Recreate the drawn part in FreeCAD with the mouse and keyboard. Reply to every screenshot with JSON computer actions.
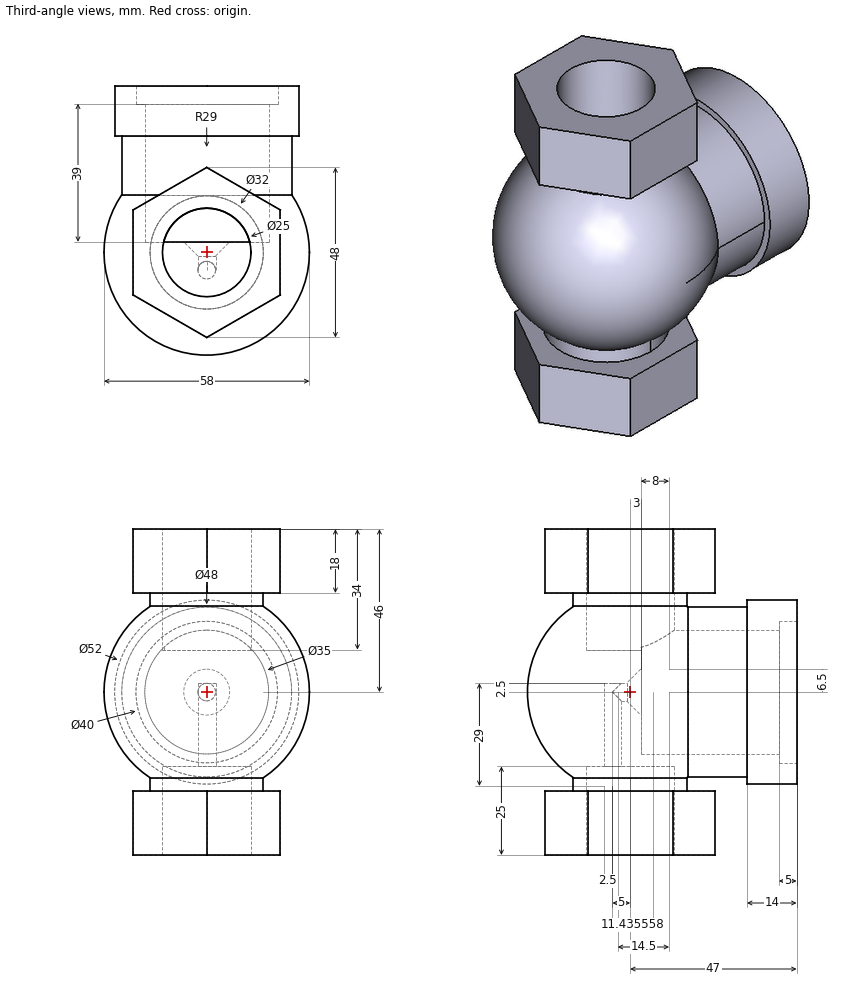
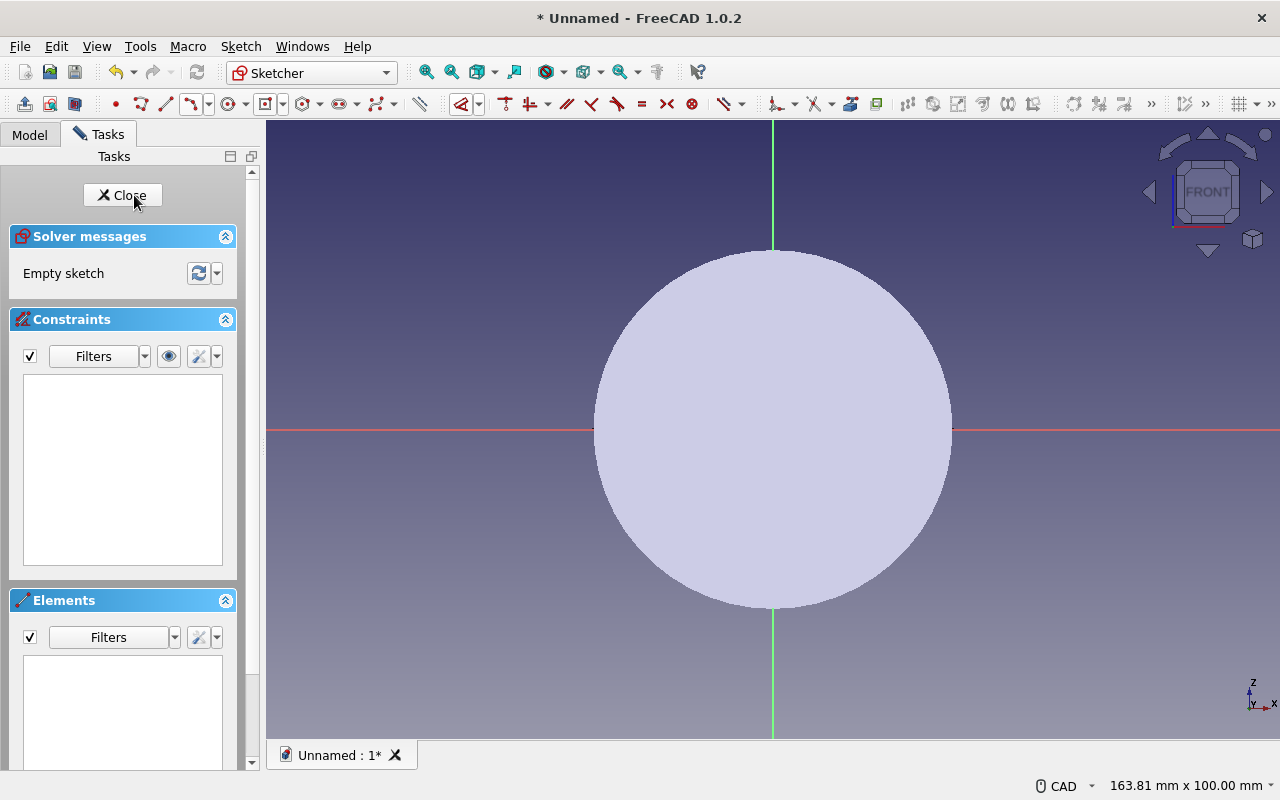
{"action": "left_click", "coordinate": [75, 104]}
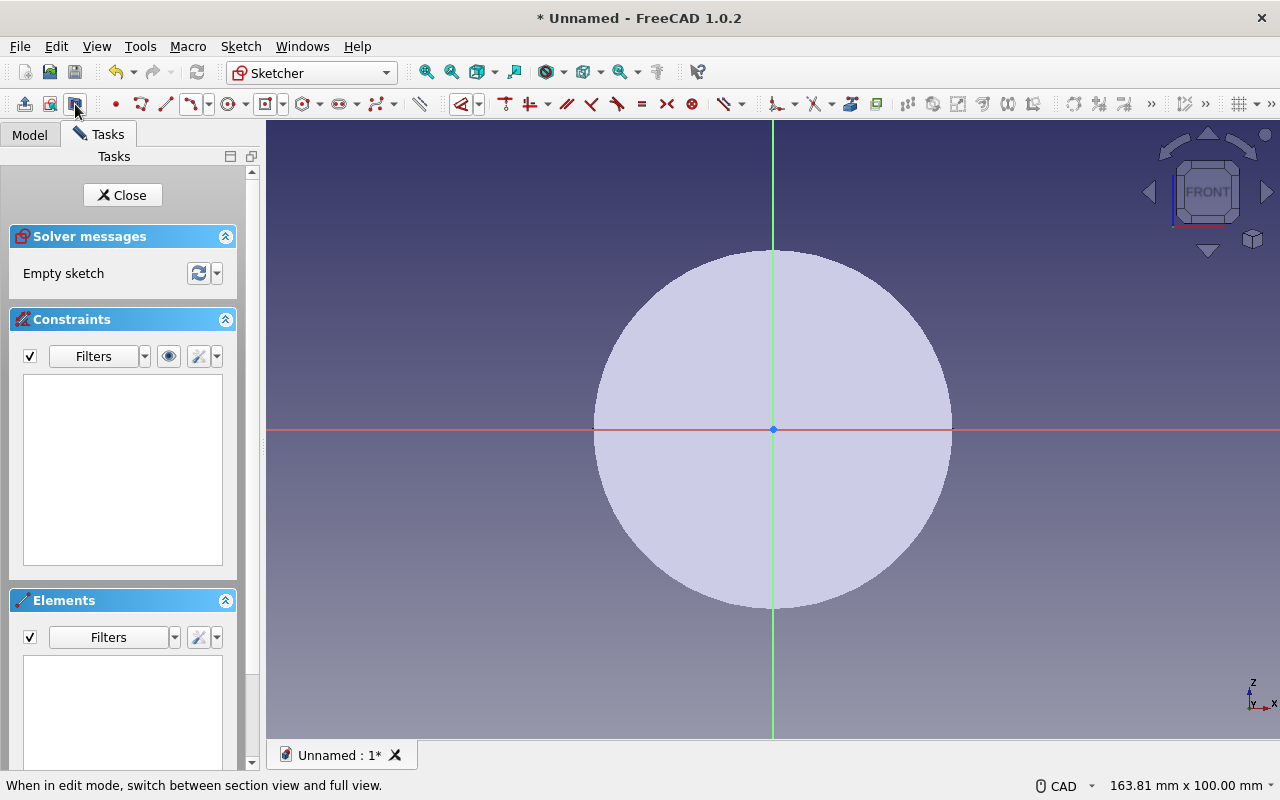
{"action": "left_click", "coordinate": [228, 104]}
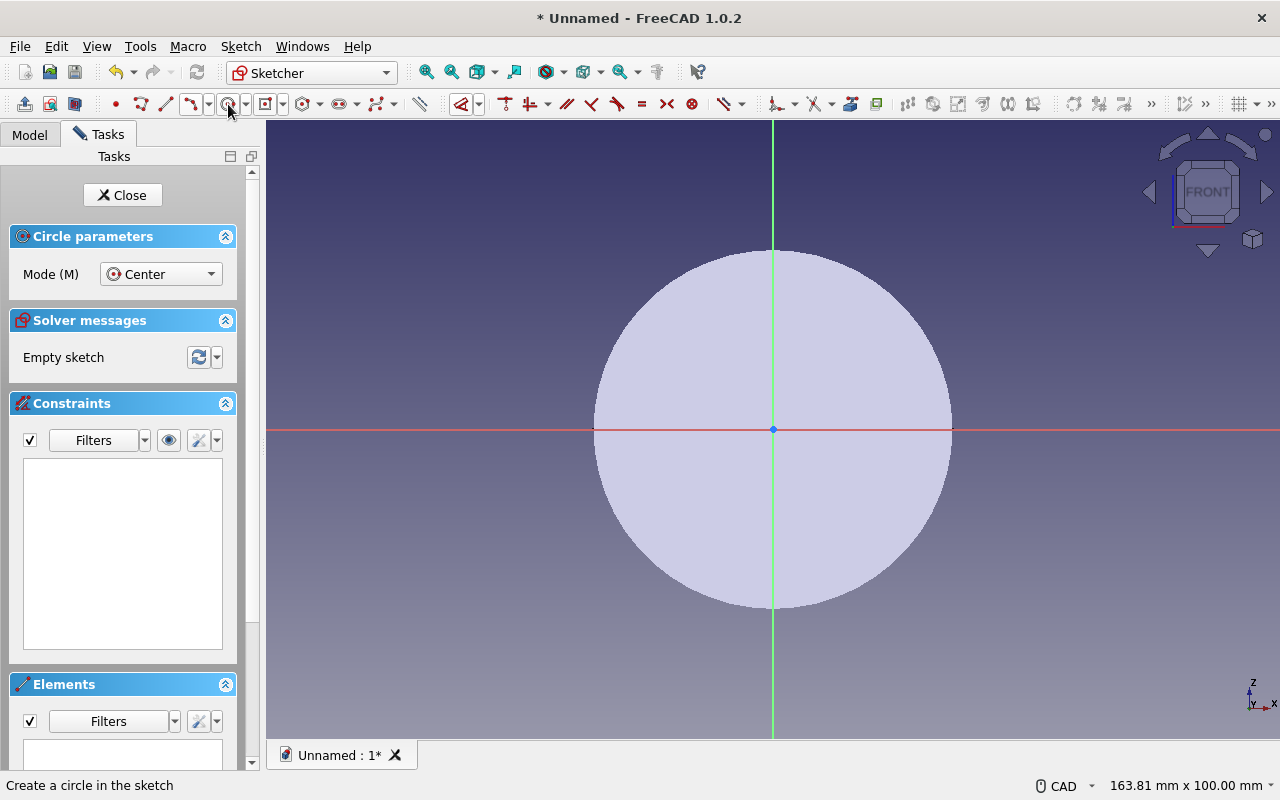
{"action": "left_click", "coordinate": [773, 430]}
{"action": "left_click", "coordinate": [878, 324]}
{"action": "key", "text": "Escape"}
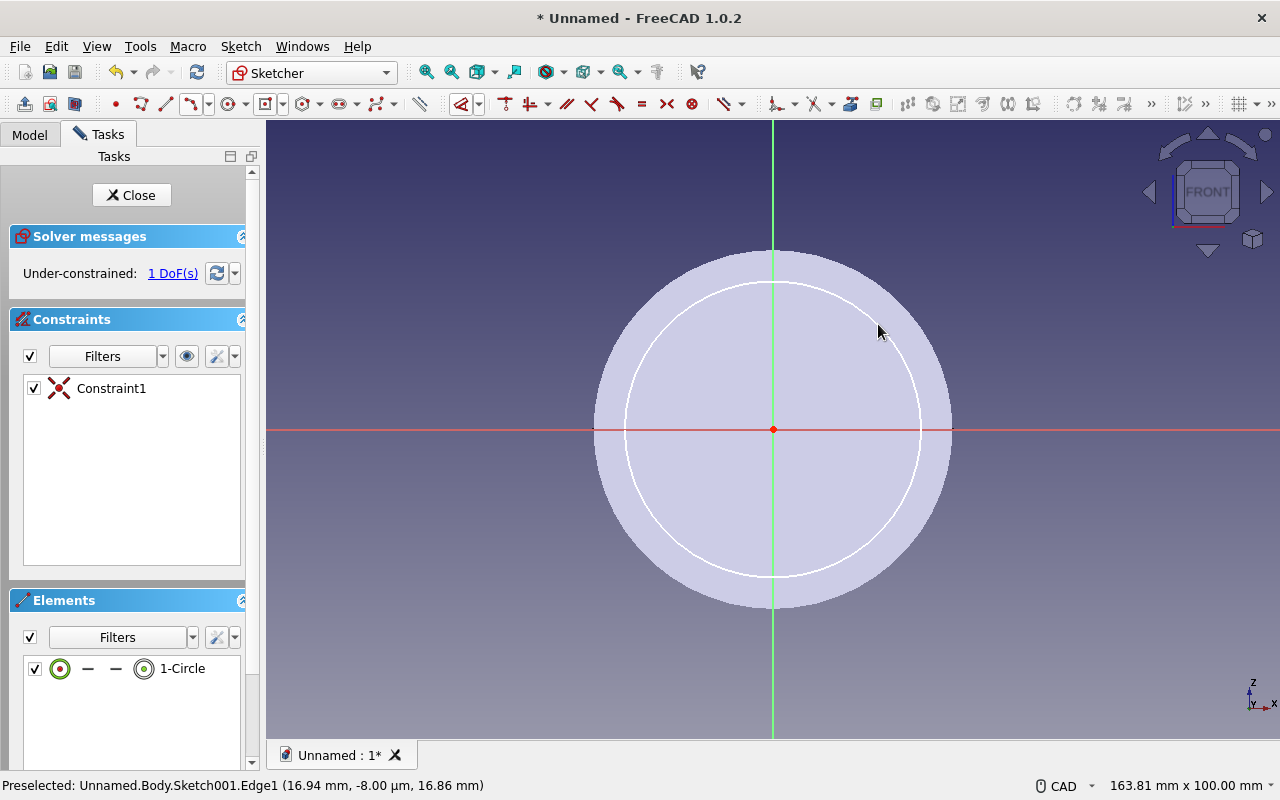
{"action": "left_click", "coordinate": [877, 324]}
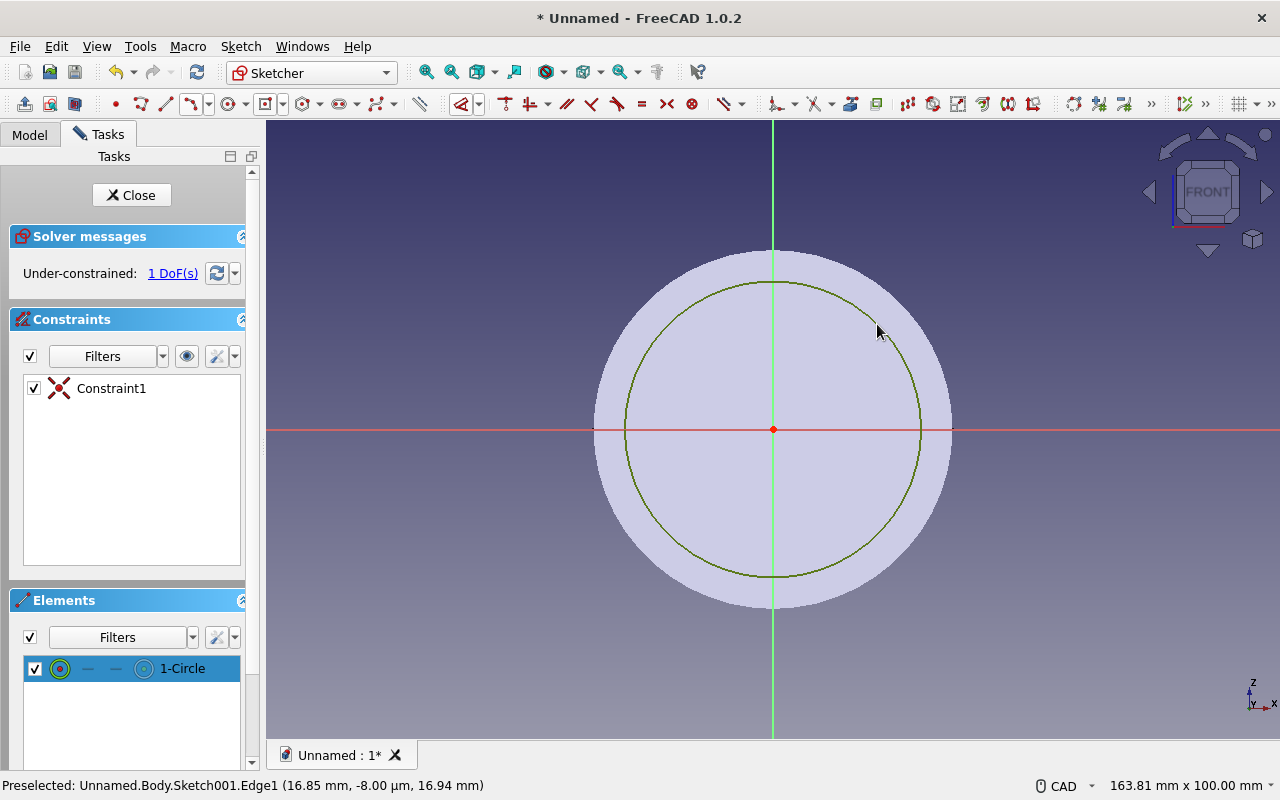
{"action": "key", "text": "k o"}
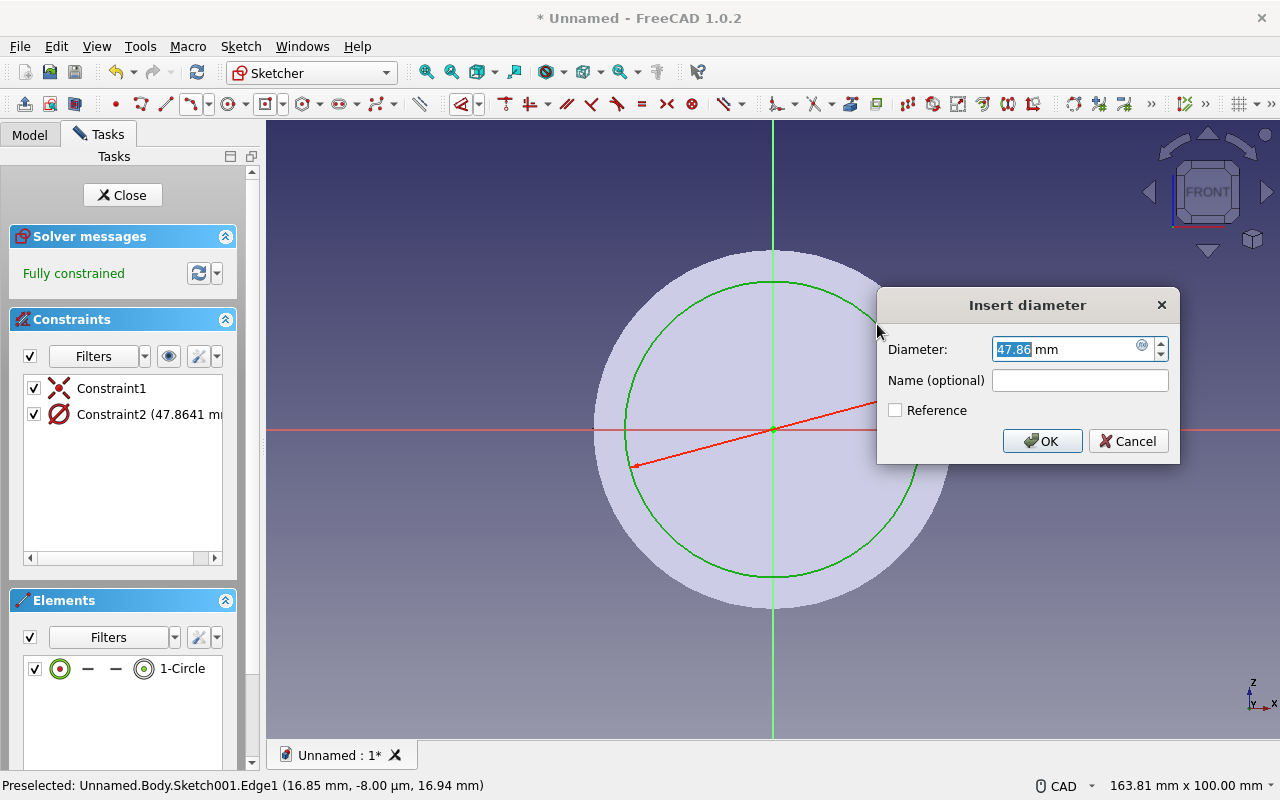
{"action": "type", "text": "48"}
{"action": "key", "text": "Return"}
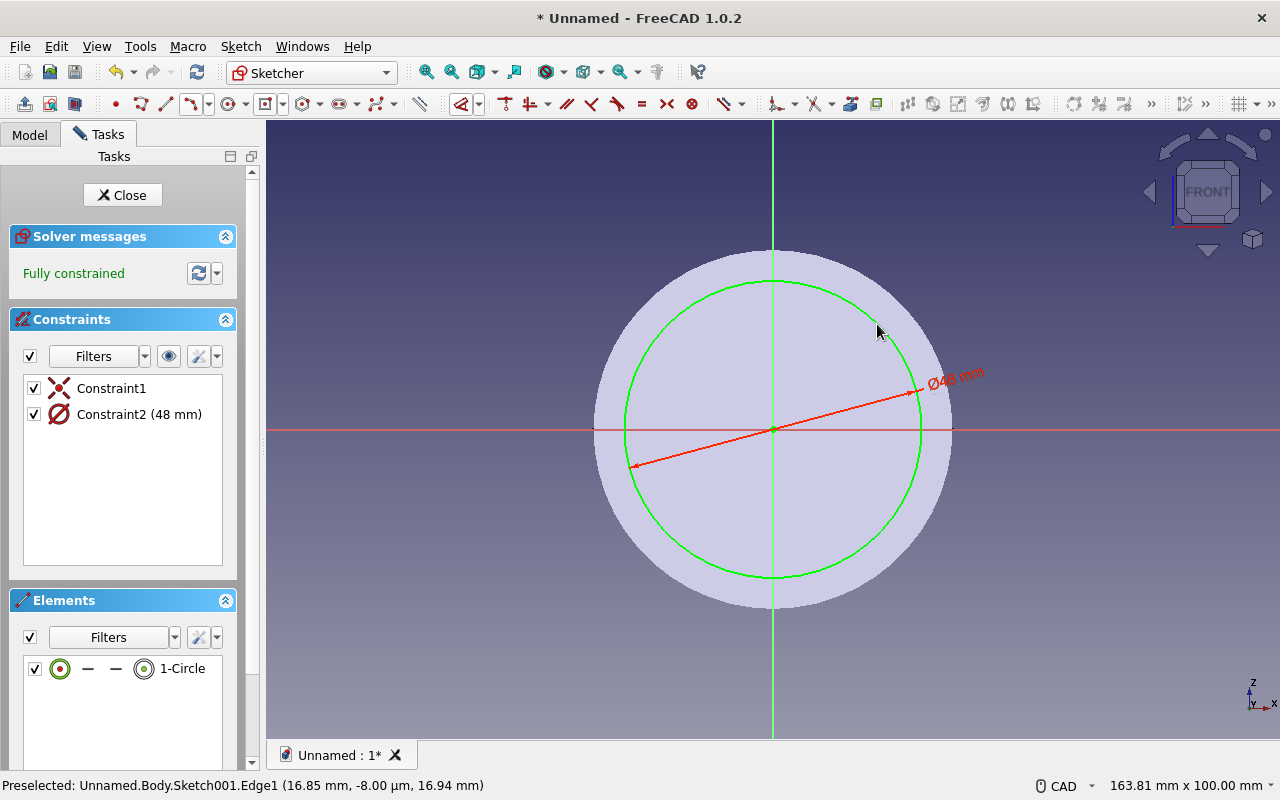
{"action": "left_click", "coordinate": [123, 195]}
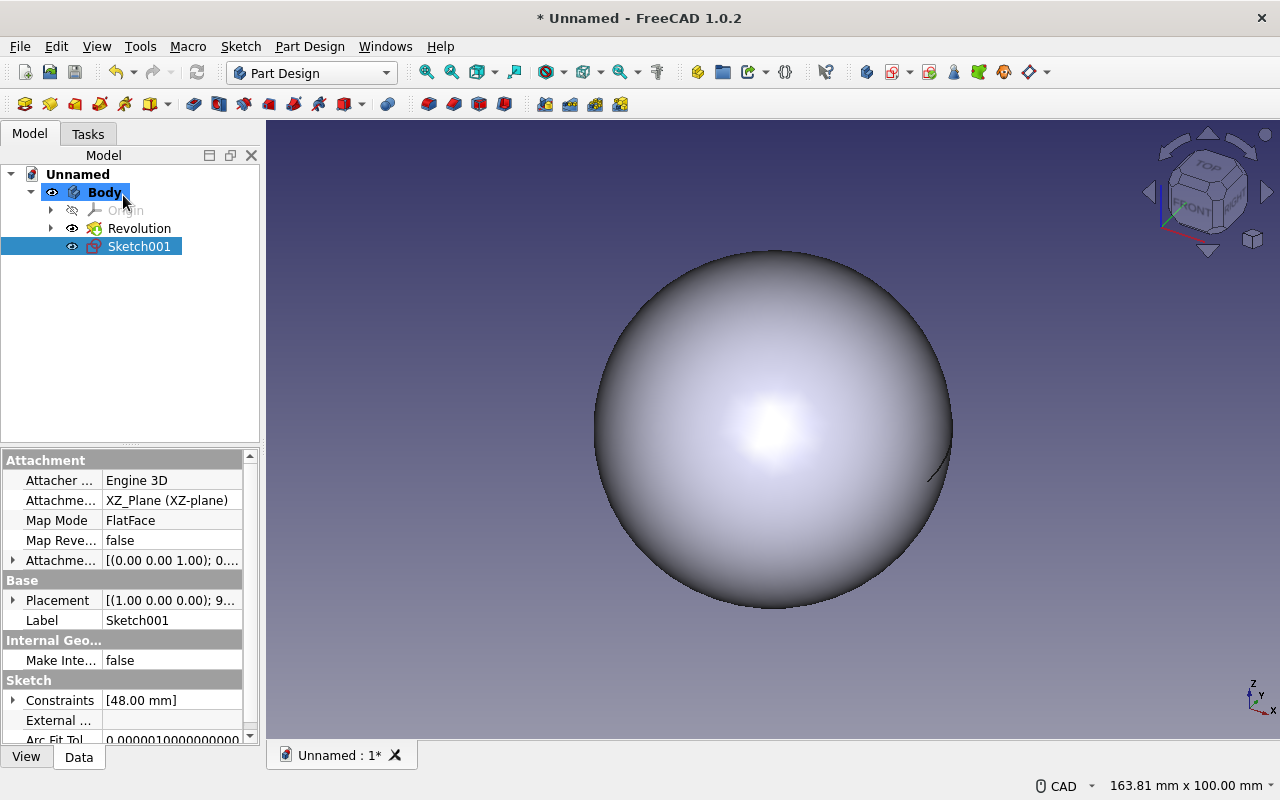
{"action": "left_click", "coordinate": [25, 104]}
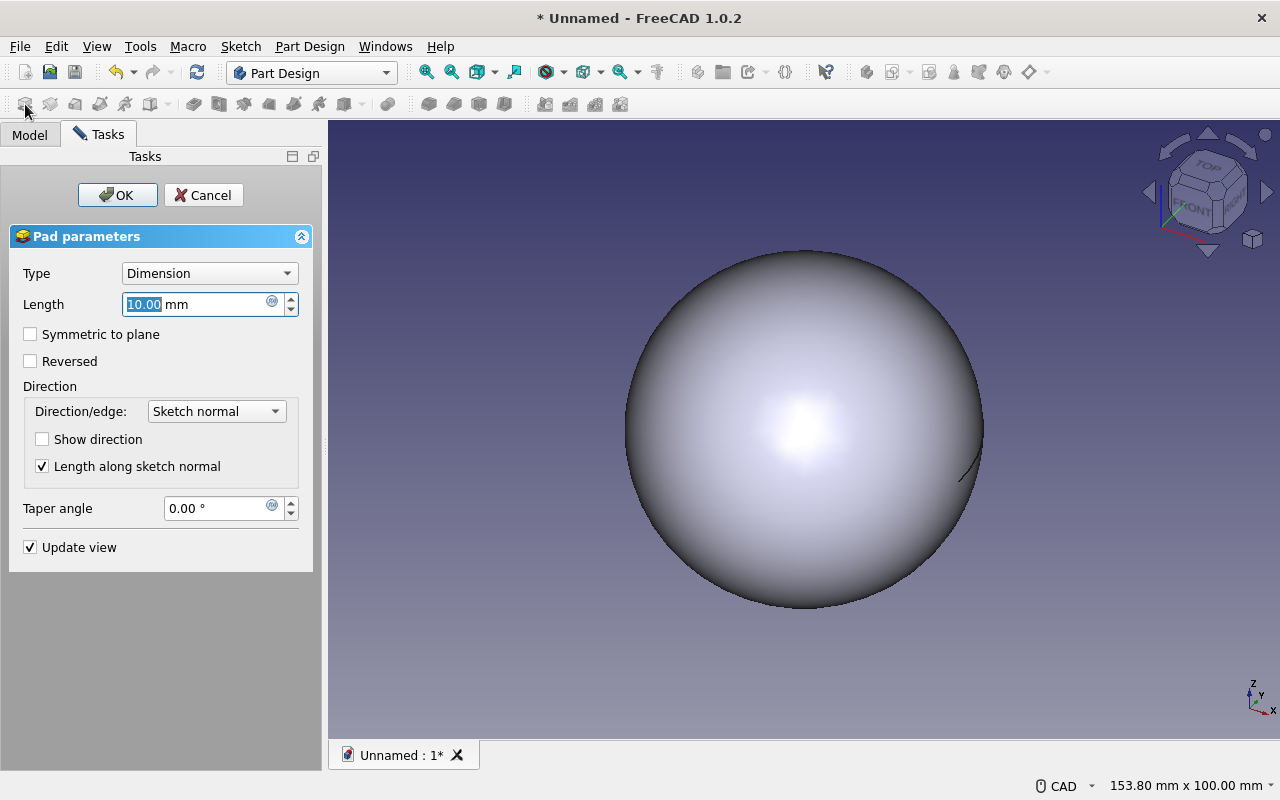
{"action": "type", "text": "47"}
{"action": "key", "text": "Tab"}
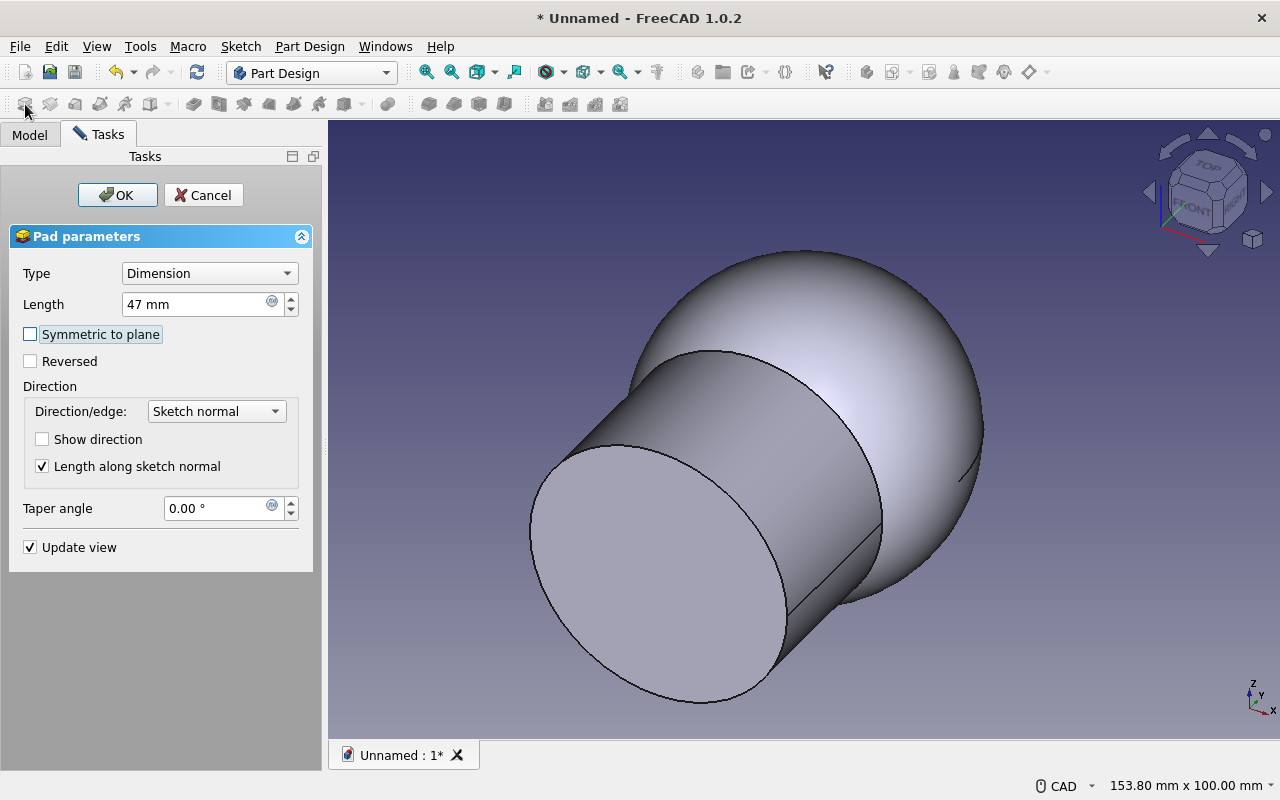
{"action": "left_click", "coordinate": [31, 361]}